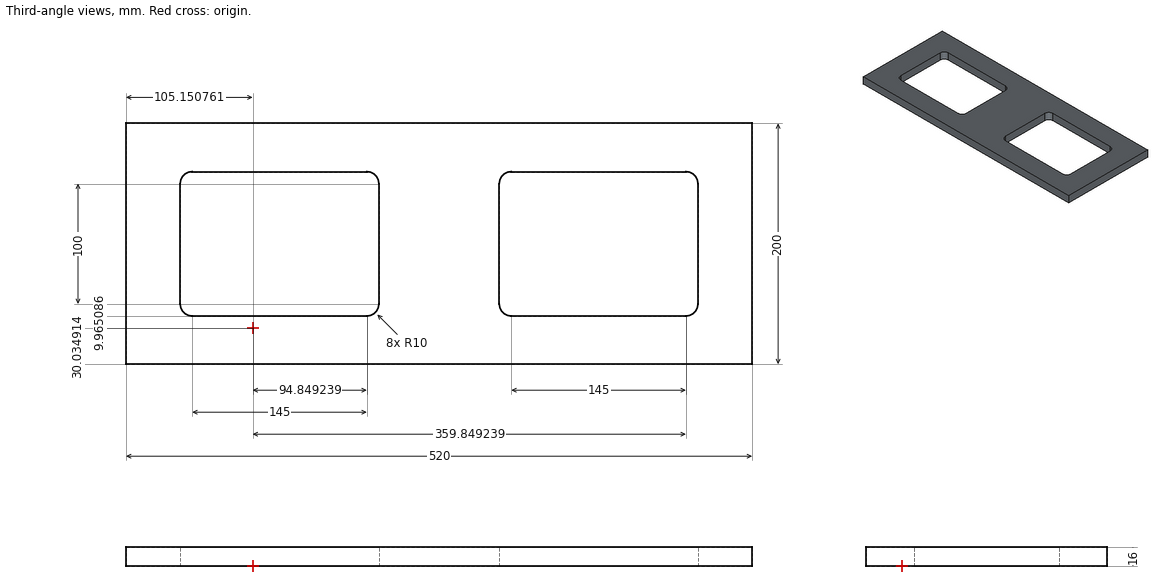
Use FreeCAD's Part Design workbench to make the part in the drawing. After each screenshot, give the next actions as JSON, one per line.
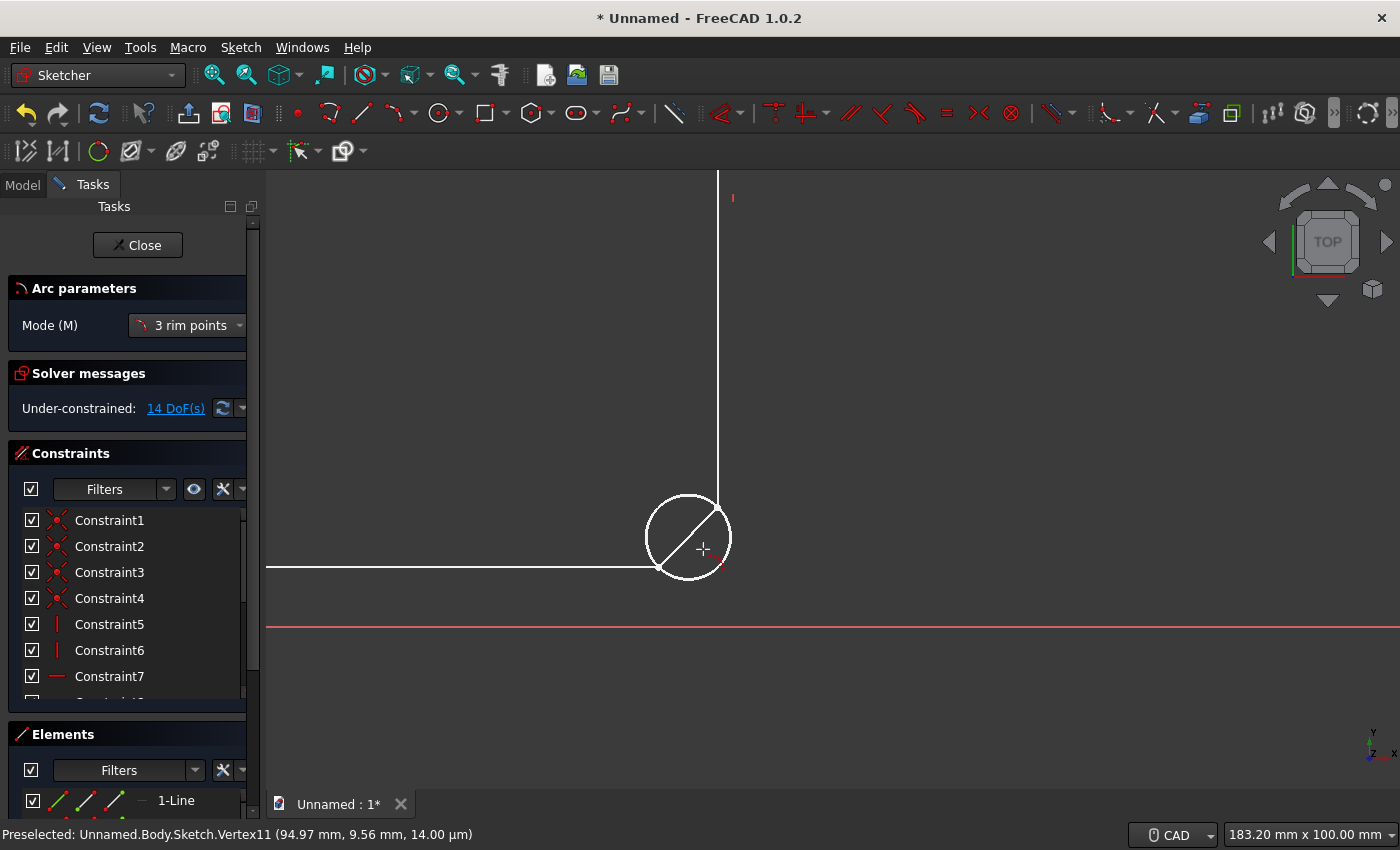
{"action": "left_click", "coordinate": [702, 547]}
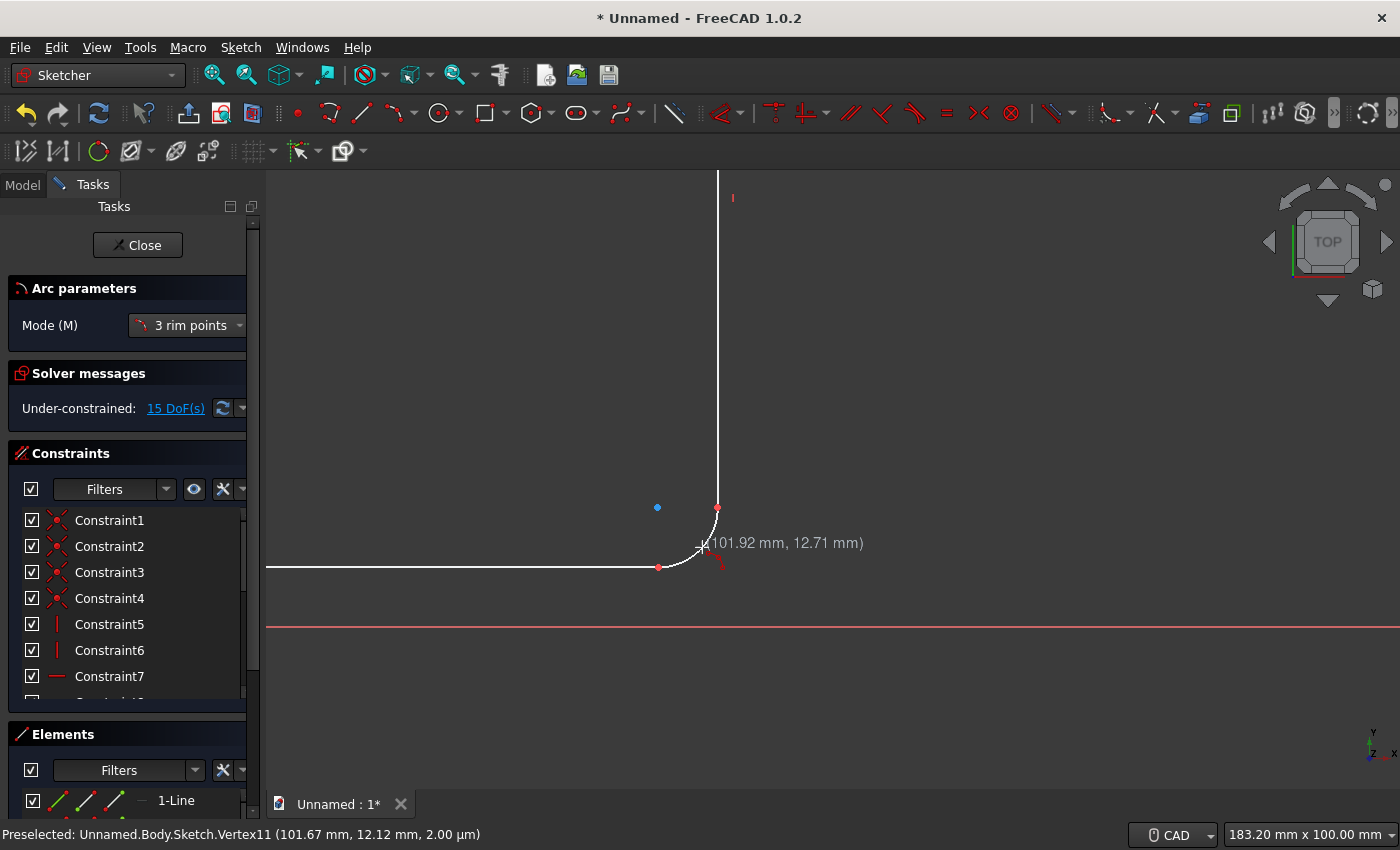
{"action": "scroll", "coordinate": [697, 552], "scroll_direction": "down", "scroll_amount": 8}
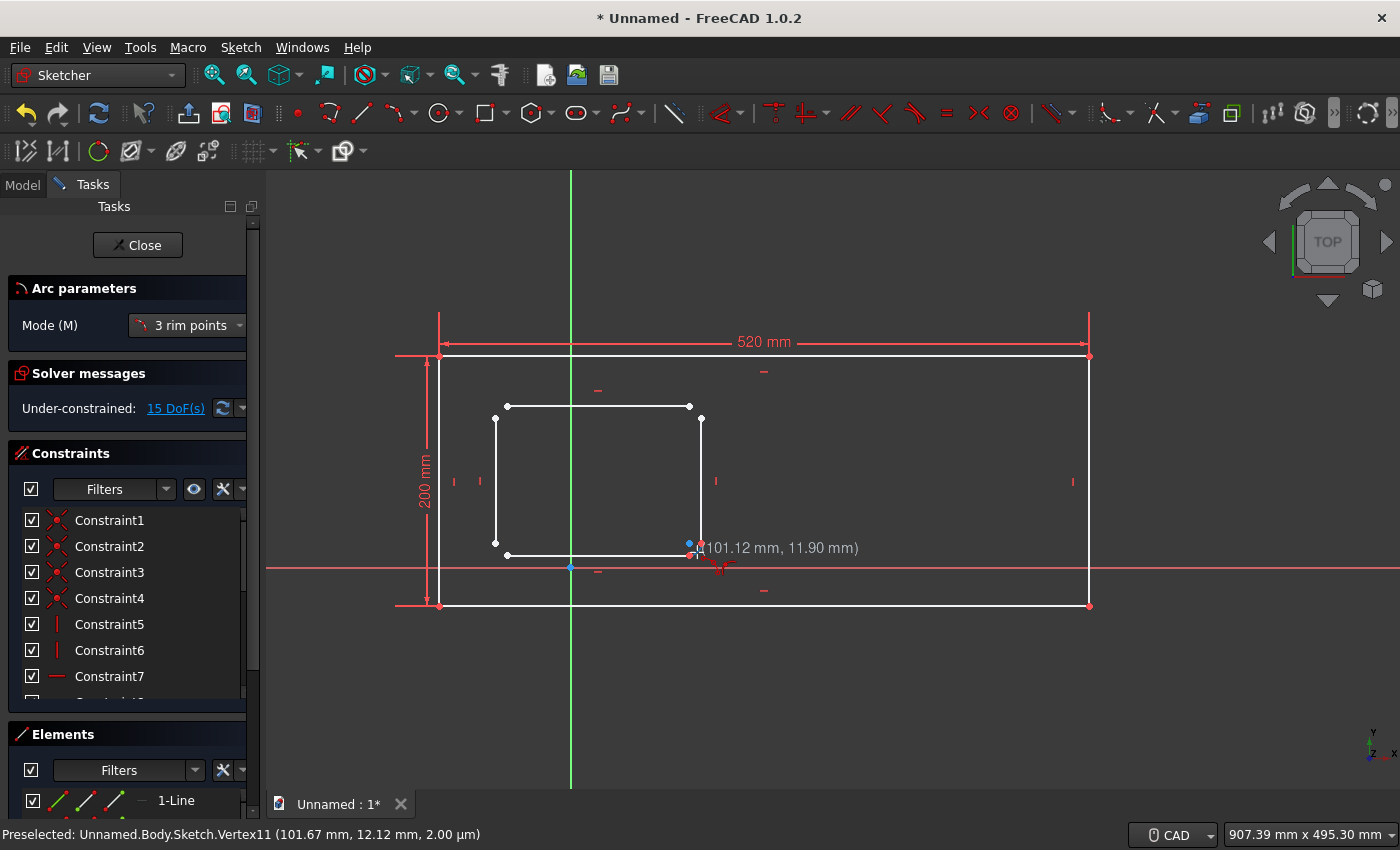
{"action": "scroll", "coordinate": [508, 555], "scroll_direction": "up", "scroll_amount": 2}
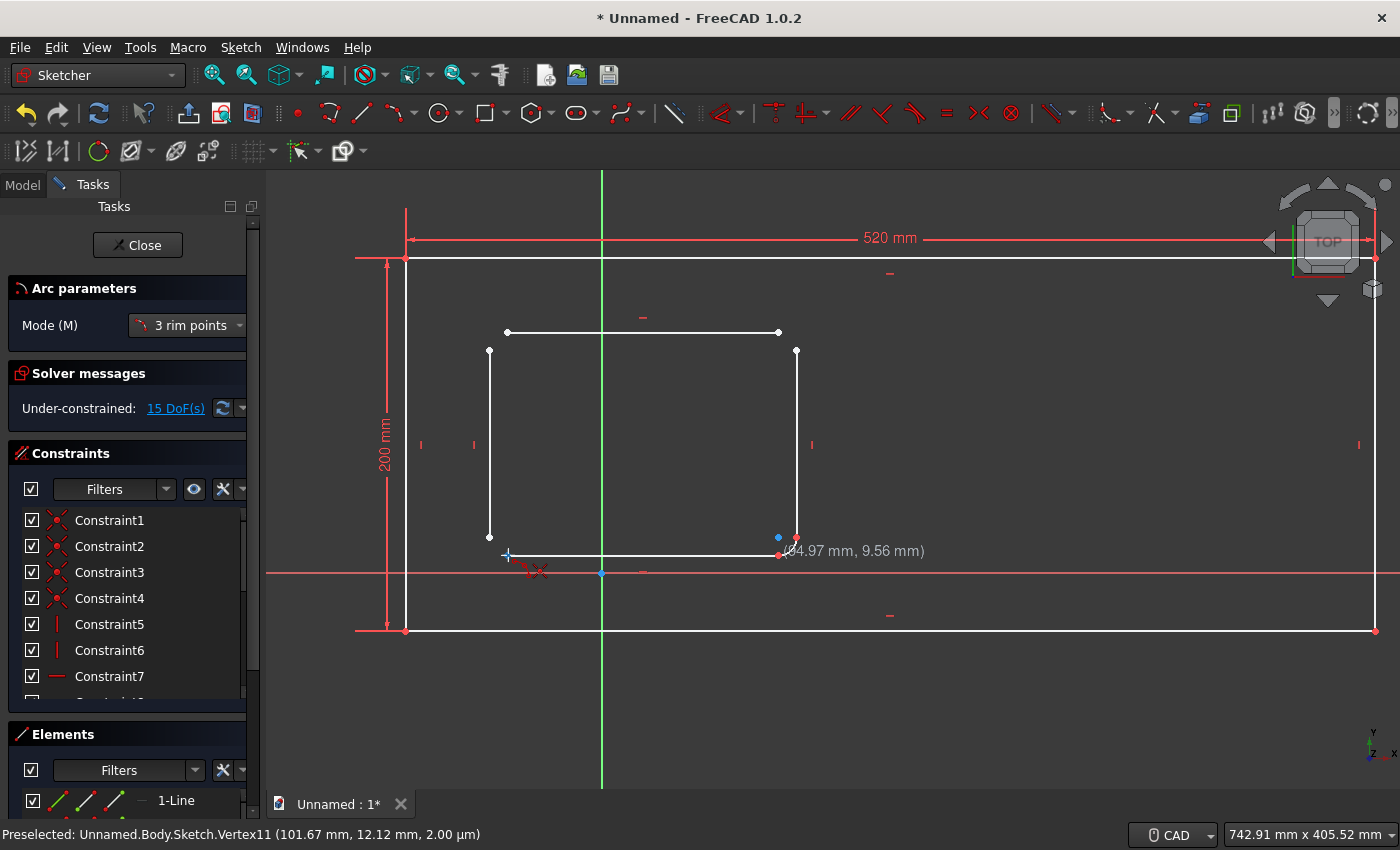
{"action": "left_click", "coordinate": [508, 556]}
{"action": "left_click", "coordinate": [490, 538]}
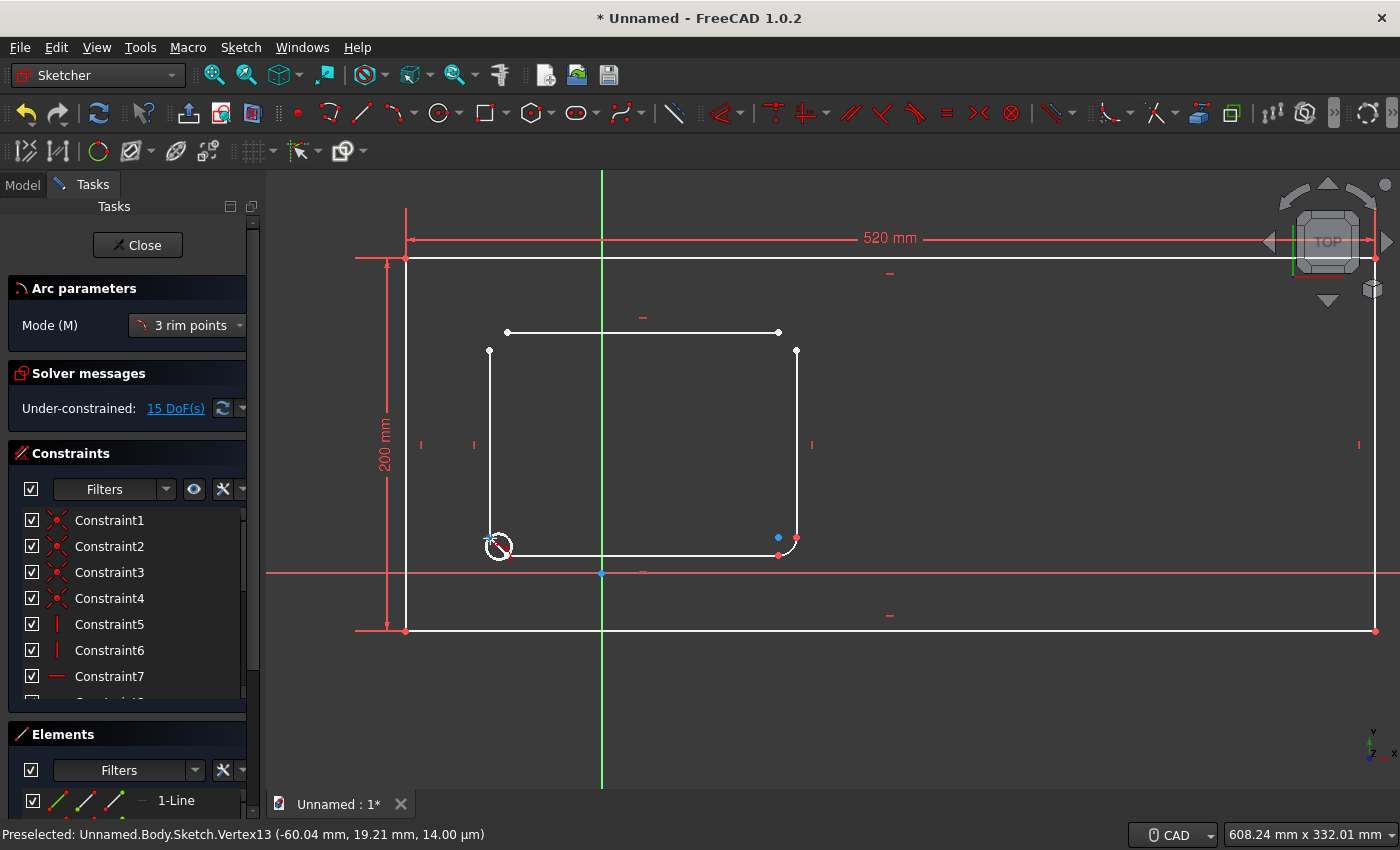
{"action": "scroll", "coordinate": [495, 549], "scroll_direction": "up", "scroll_amount": 6}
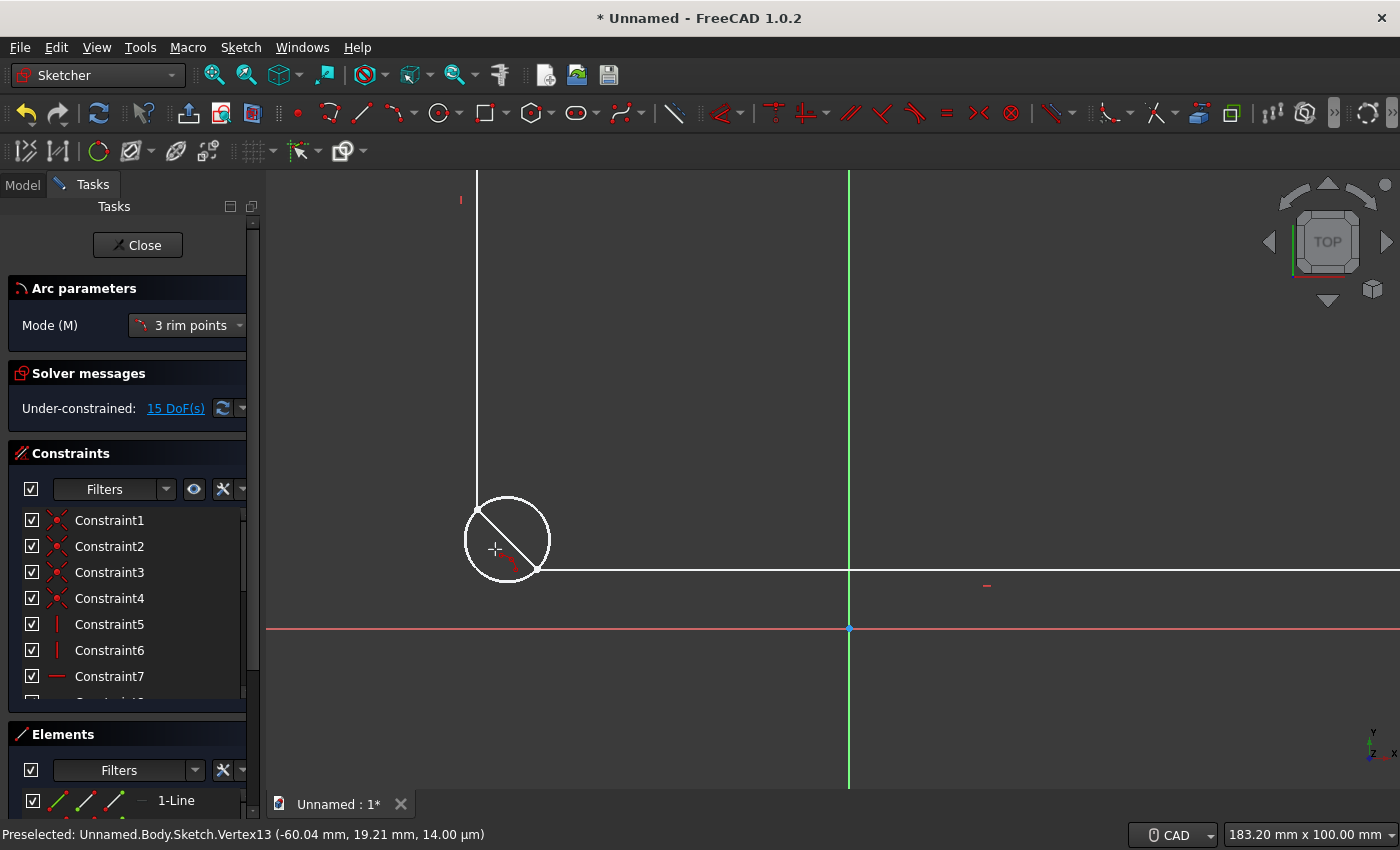
{"action": "left_click", "coordinate": [495, 549]}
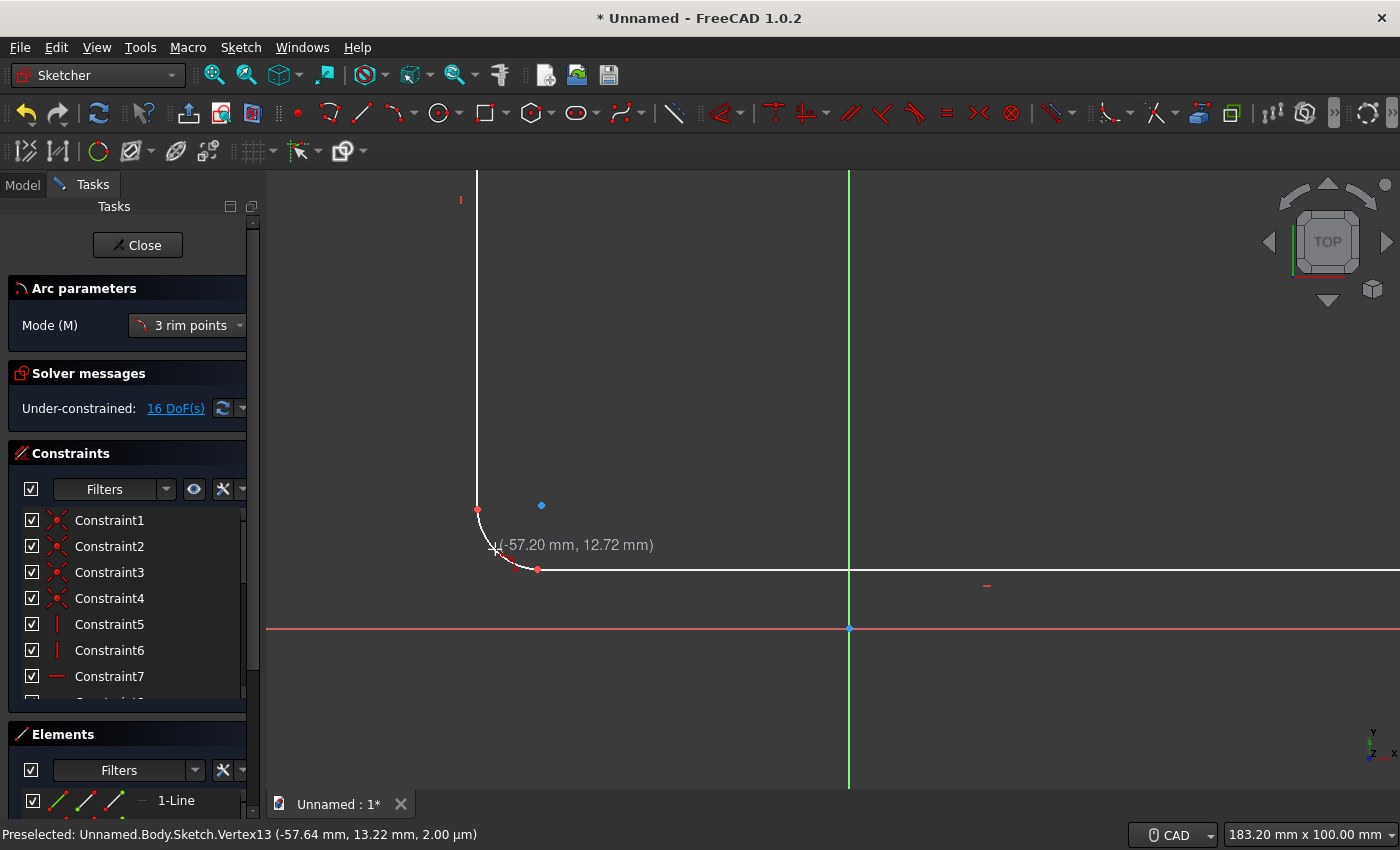
{"action": "scroll", "coordinate": [501, 551], "scroll_direction": "down", "scroll_amount": 8}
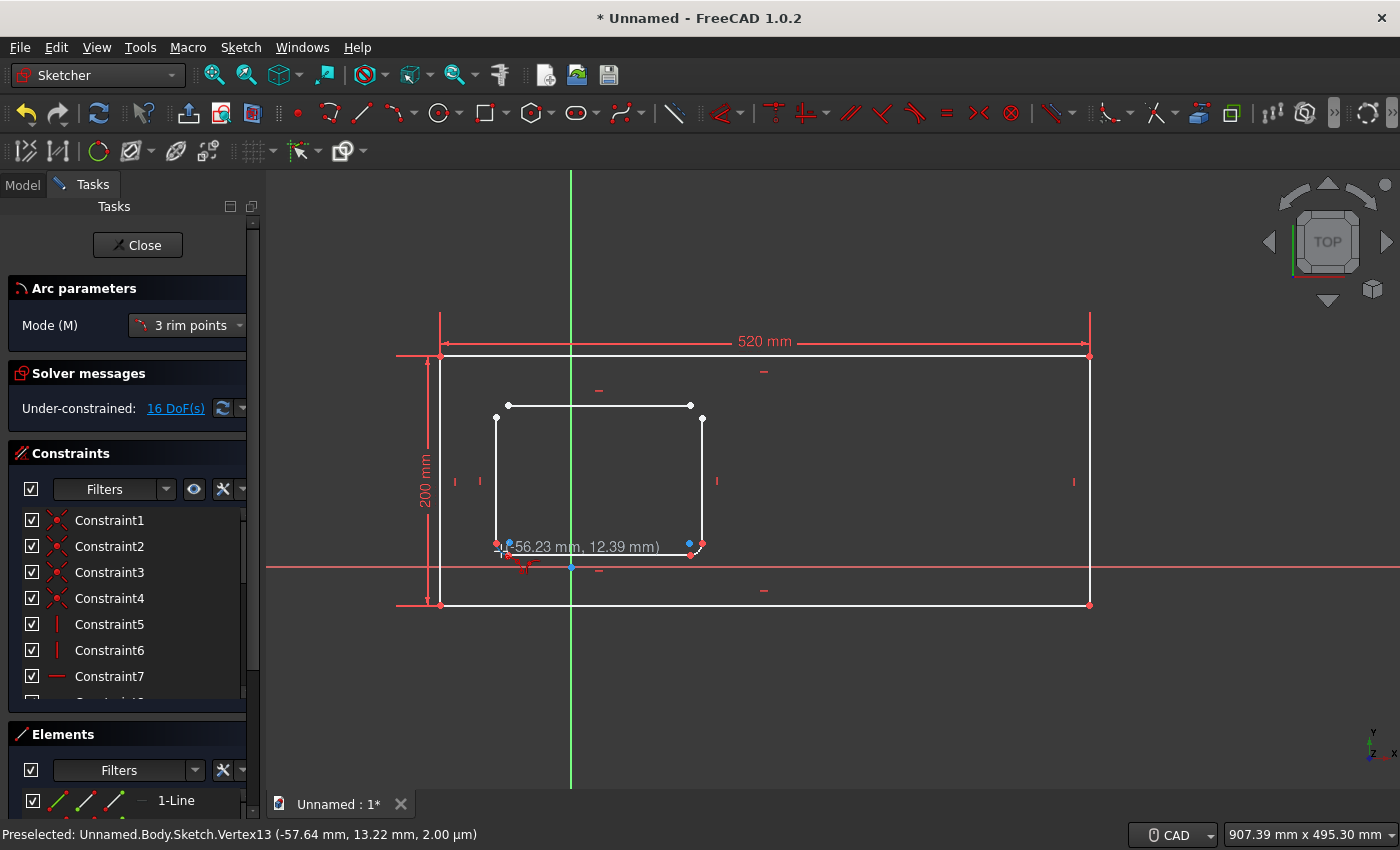
{"action": "left_click", "coordinate": [496, 418]}
{"action": "left_click", "coordinate": [508, 406]}